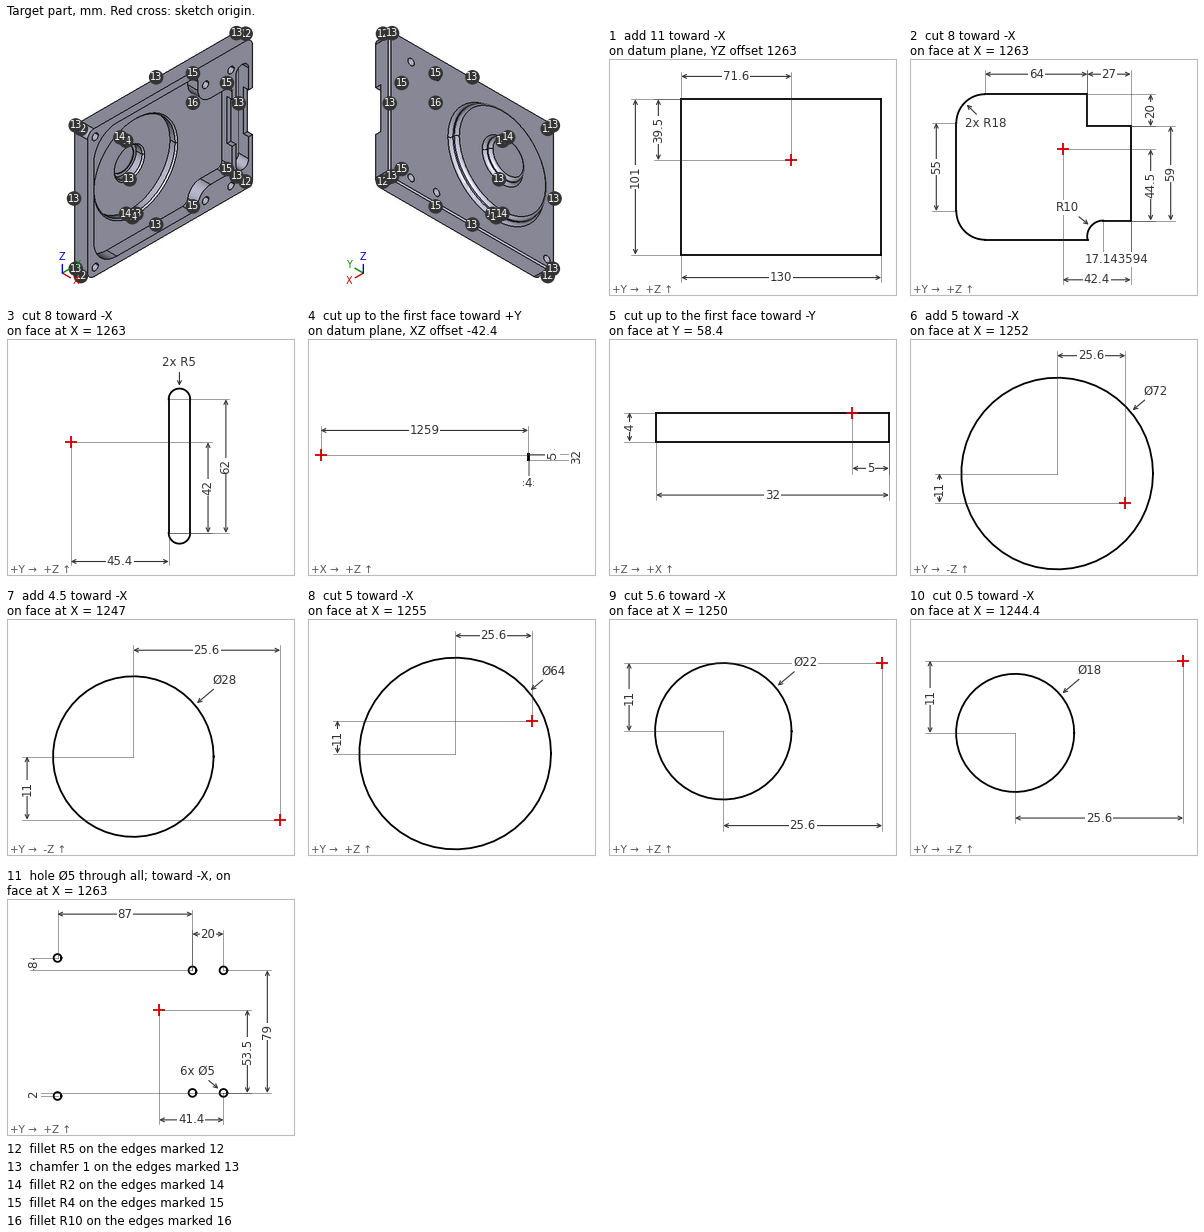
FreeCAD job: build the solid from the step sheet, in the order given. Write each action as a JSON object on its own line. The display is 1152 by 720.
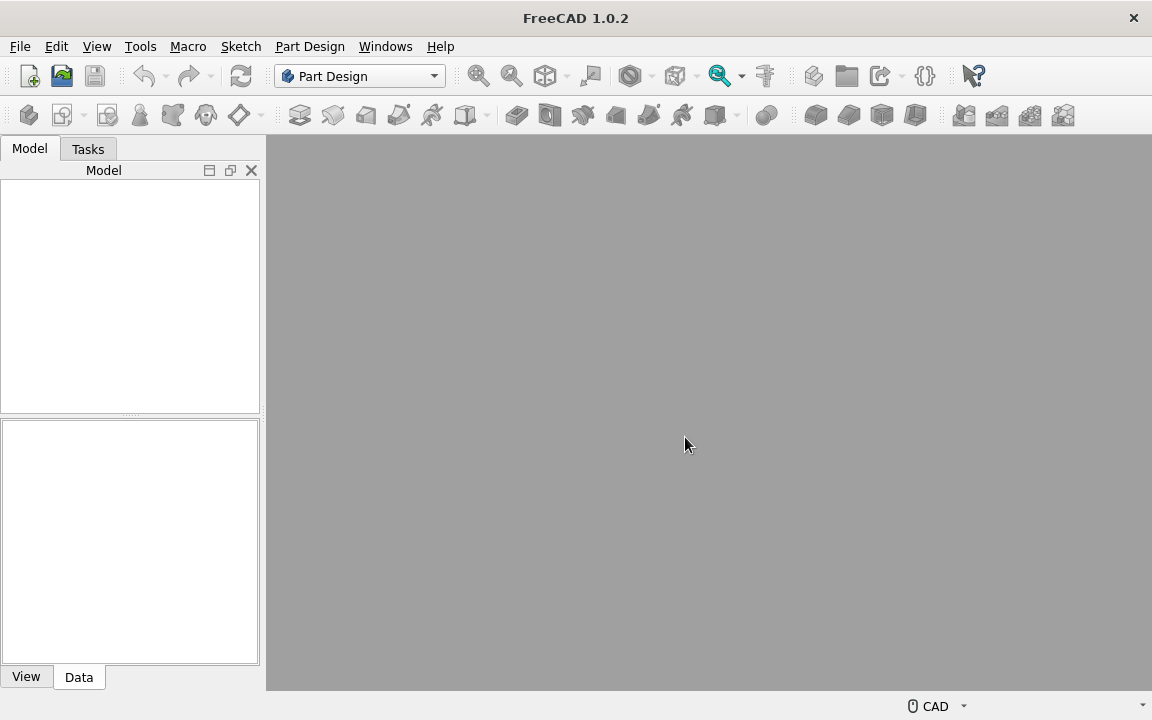
{"action": "left_click", "coordinate": [29, 76]}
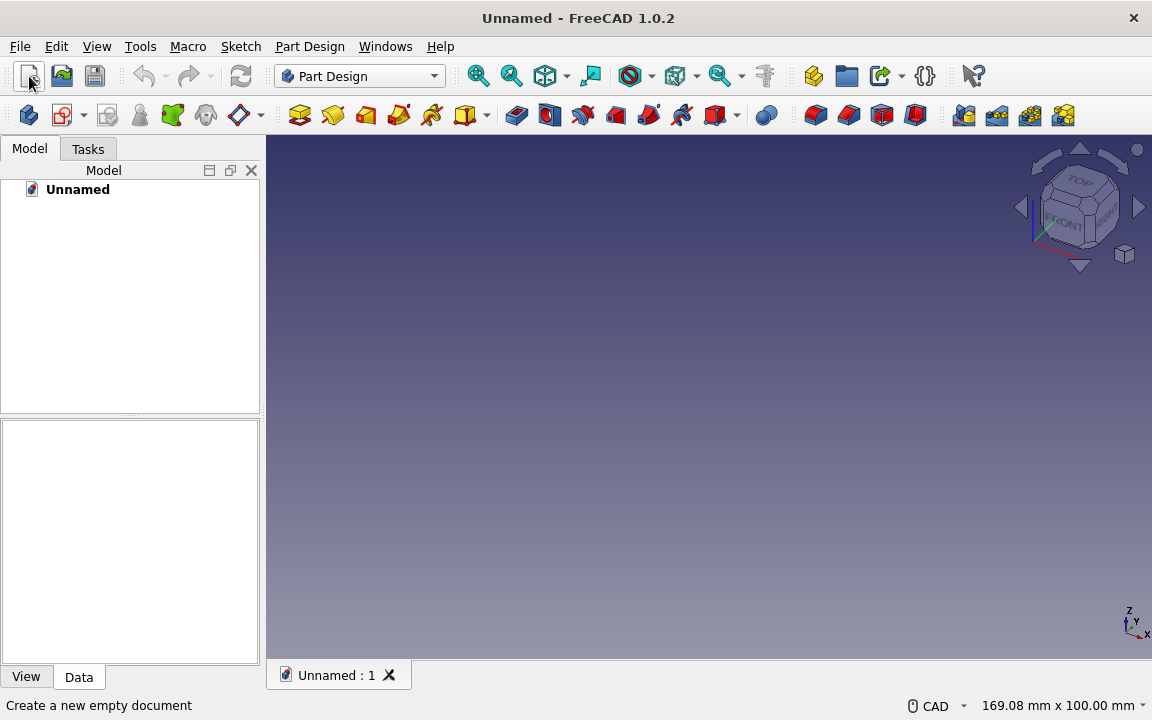
{"action": "left_click", "coordinate": [29, 116]}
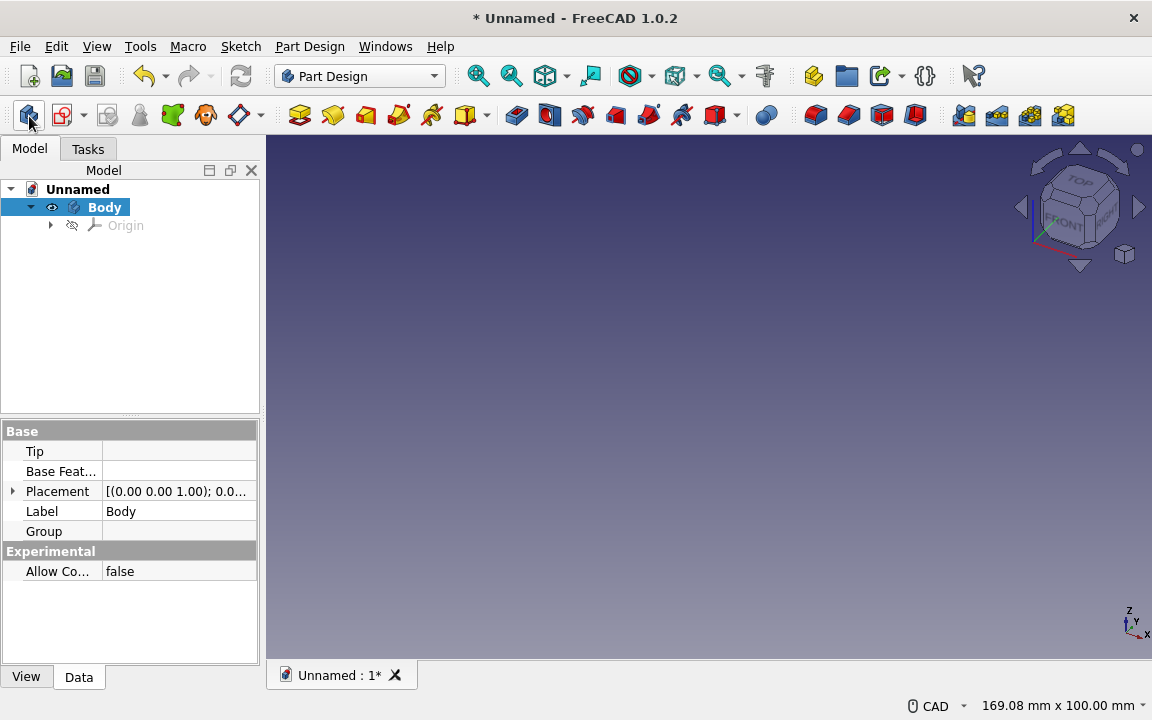
{"action": "left_click", "coordinate": [51, 225]}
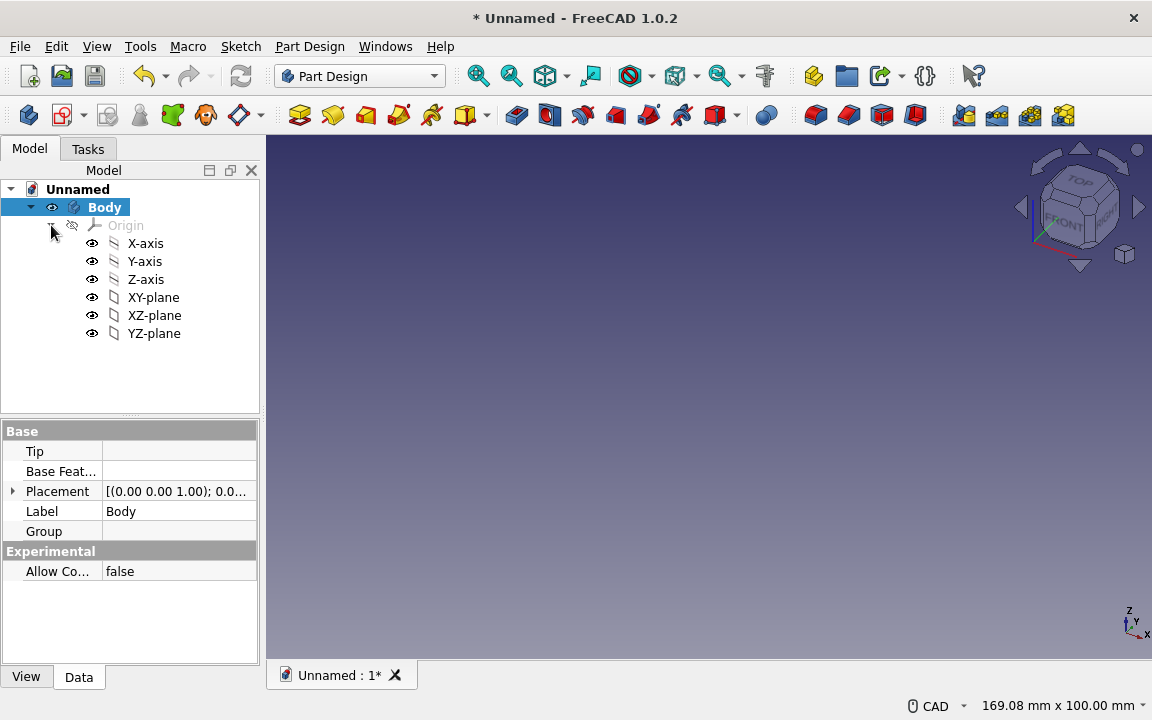
{"action": "left_click", "coordinate": [137, 333]}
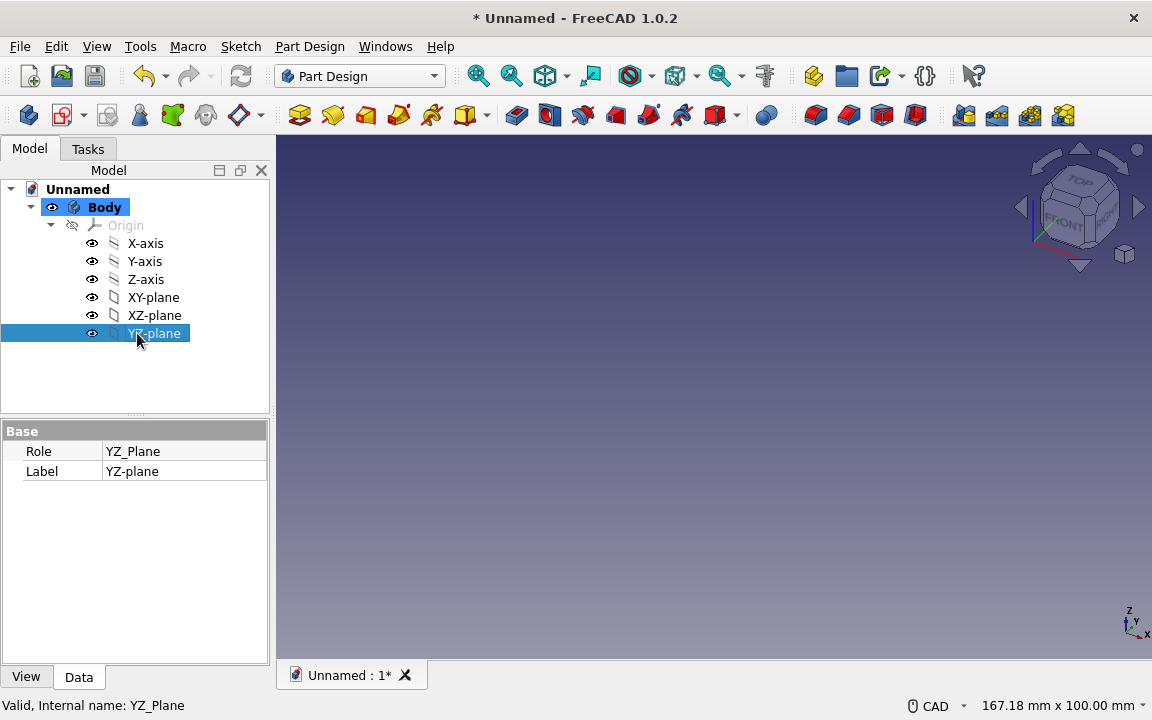
{"action": "left_click", "coordinate": [238, 116]}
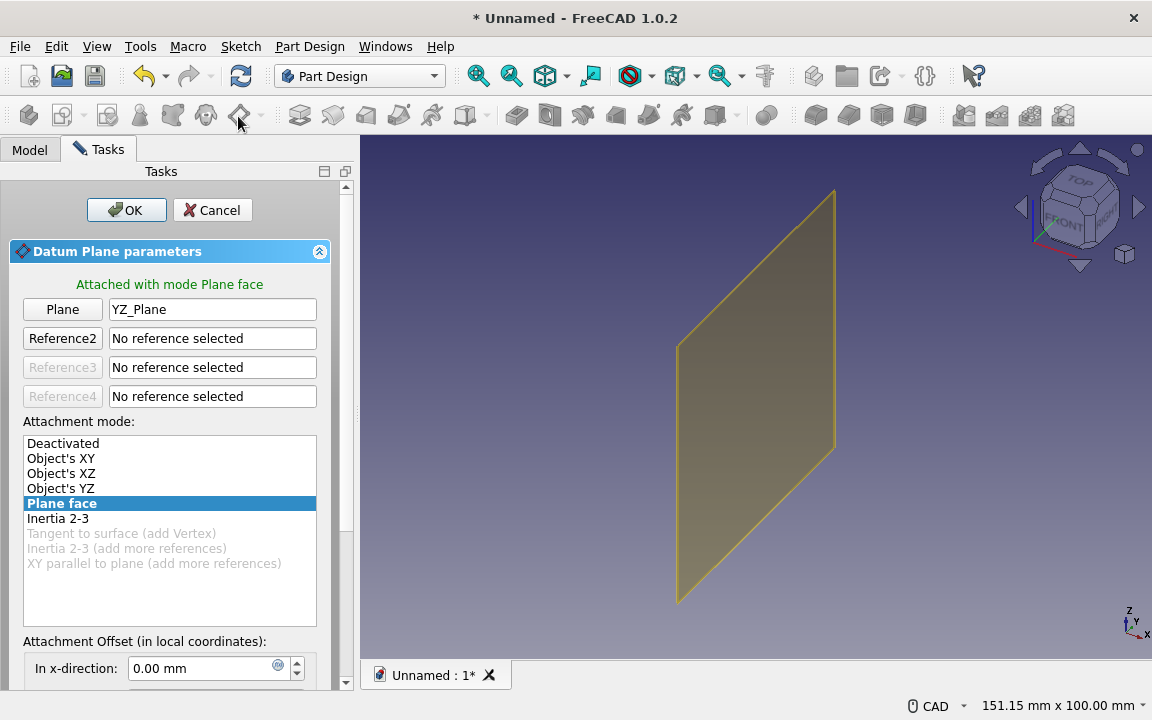
{"action": "scroll", "coordinate": [346, 436], "scroll_direction": "down", "scroll_amount": 2}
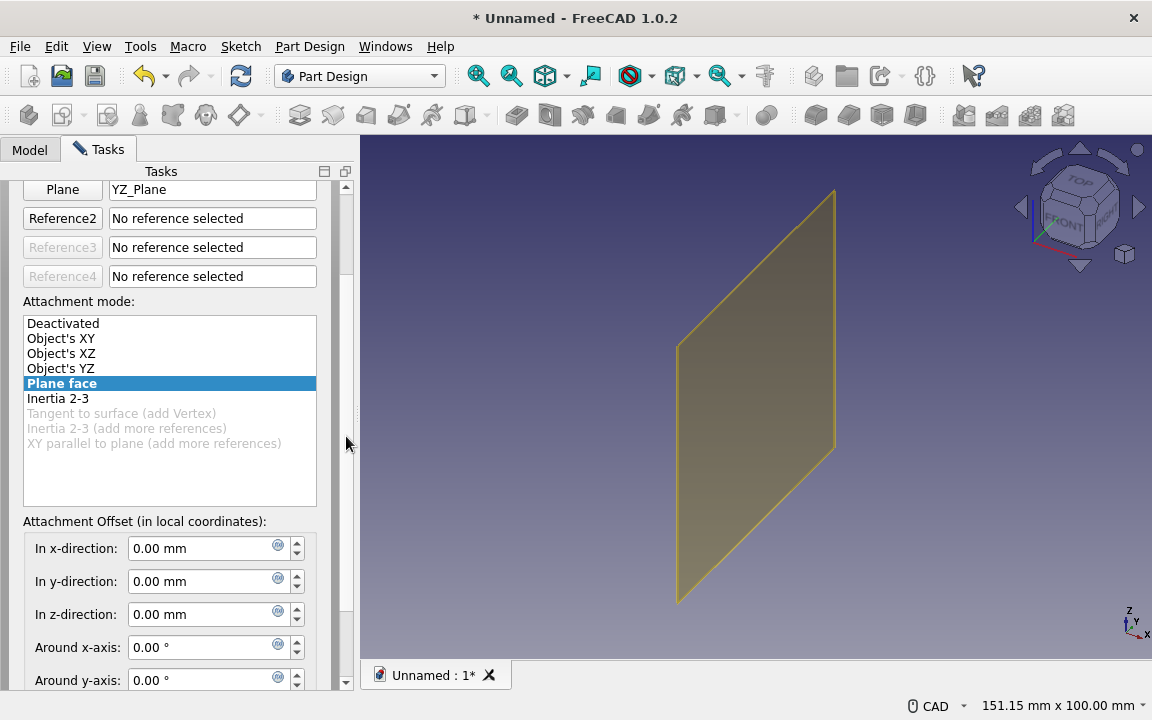
{"action": "triple_click", "coordinate": [210, 614]}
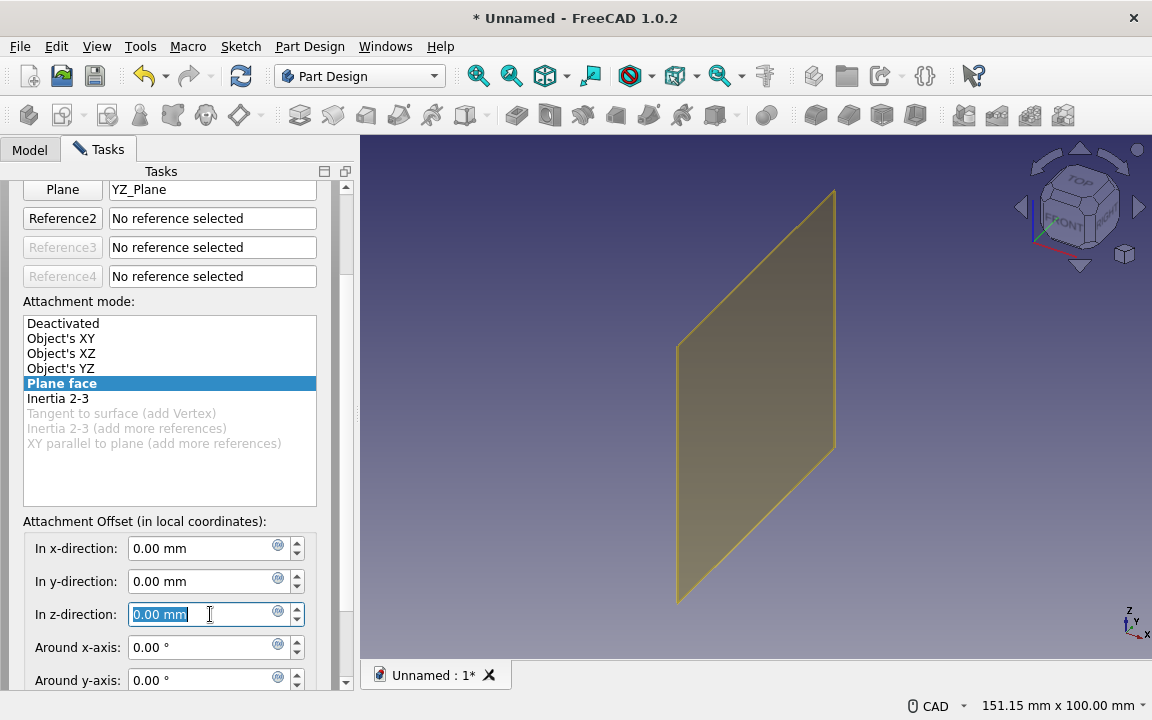
{"action": "type", "text": "1263"}
{"action": "key", "text": "Tab"}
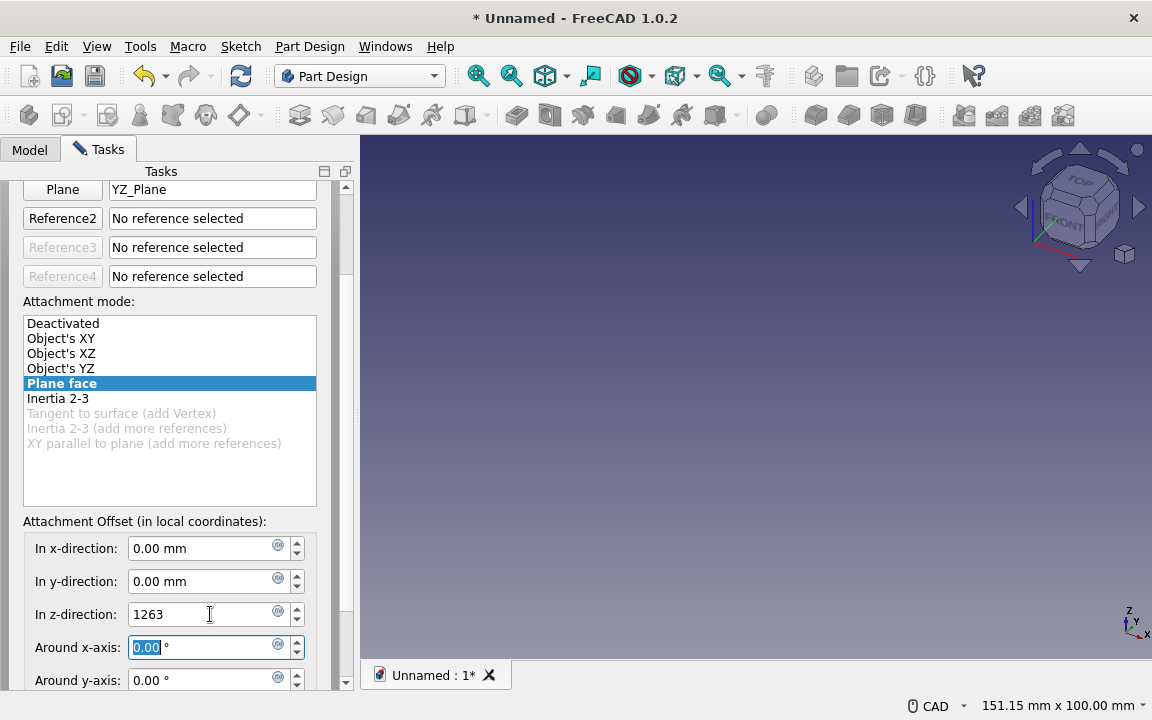
{"action": "scroll", "coordinate": [346, 436], "scroll_direction": "up", "scroll_amount": 3}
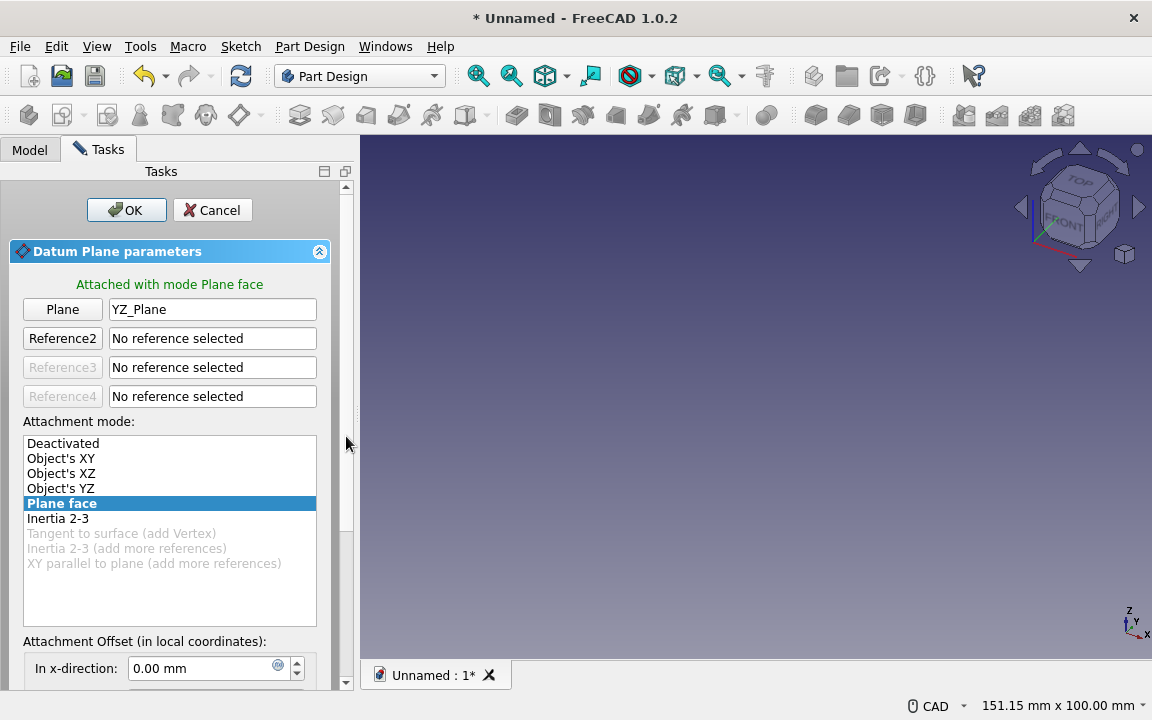
{"action": "left_click", "coordinate": [127, 210]}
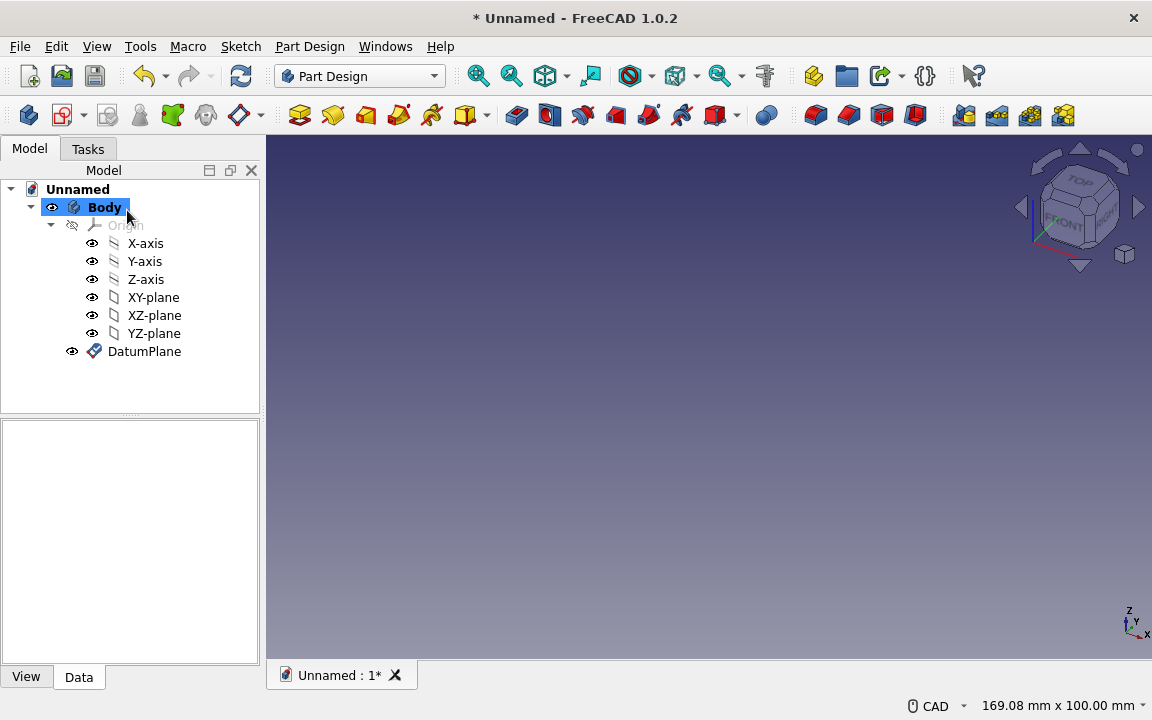
{"action": "left_click", "coordinate": [117, 351]}